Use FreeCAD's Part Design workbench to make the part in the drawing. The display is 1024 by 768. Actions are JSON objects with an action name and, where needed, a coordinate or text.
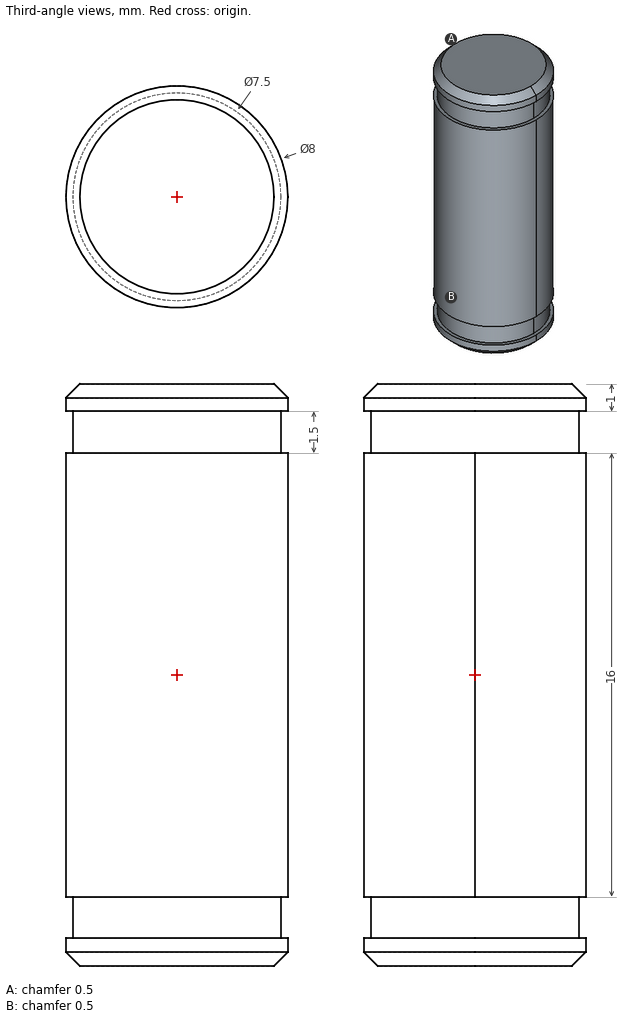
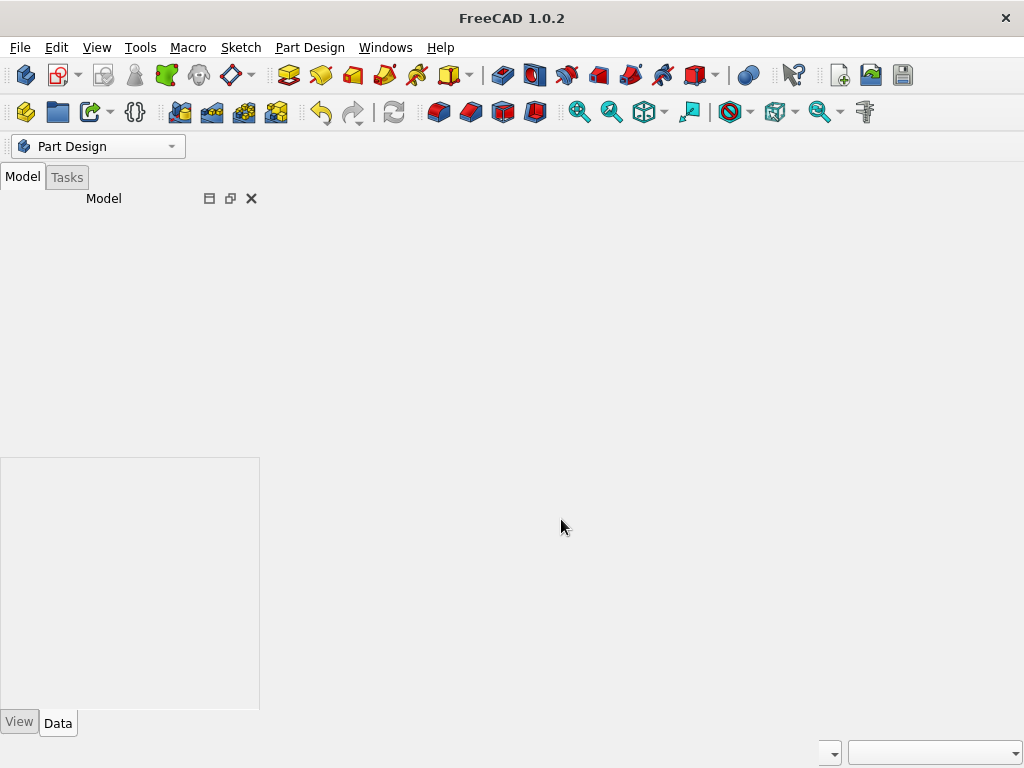
{"action": "left_click", "coordinate": [840, 76]}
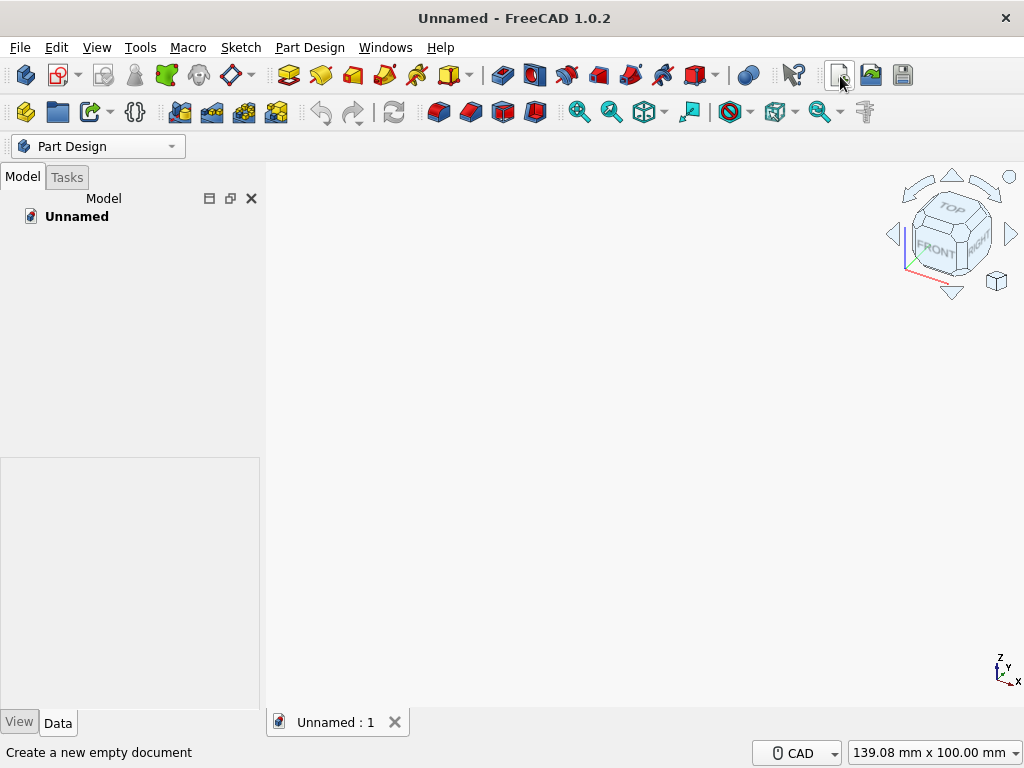
{"action": "left_click", "coordinate": [58, 76]}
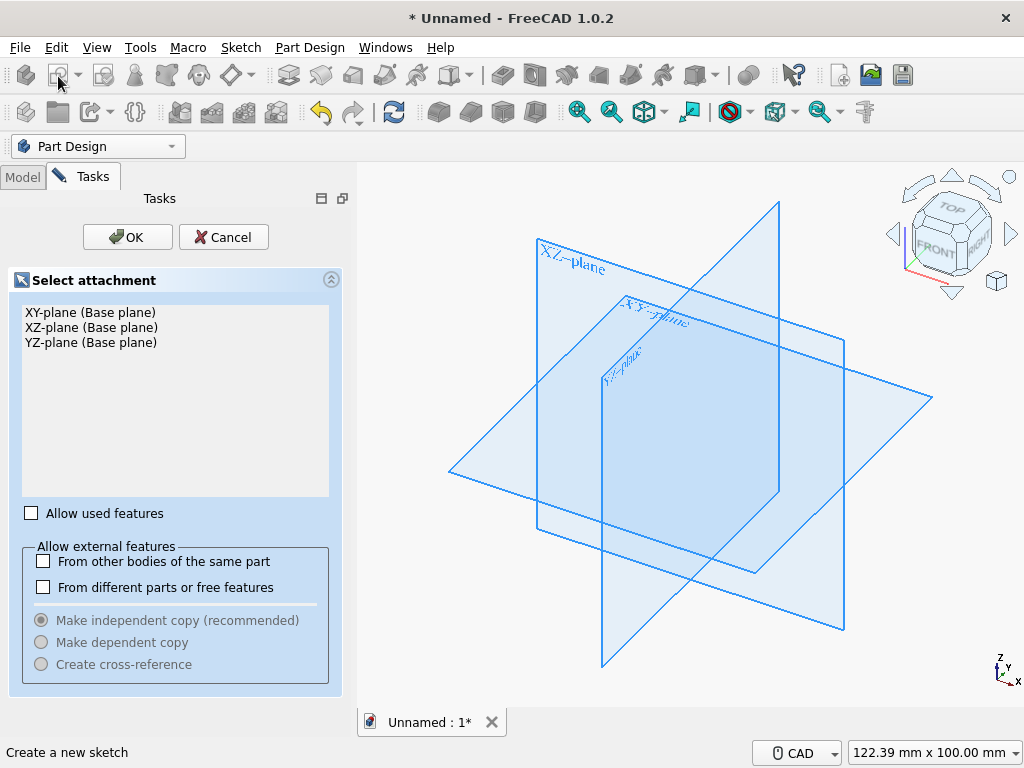
{"action": "left_click", "coordinate": [82, 312]}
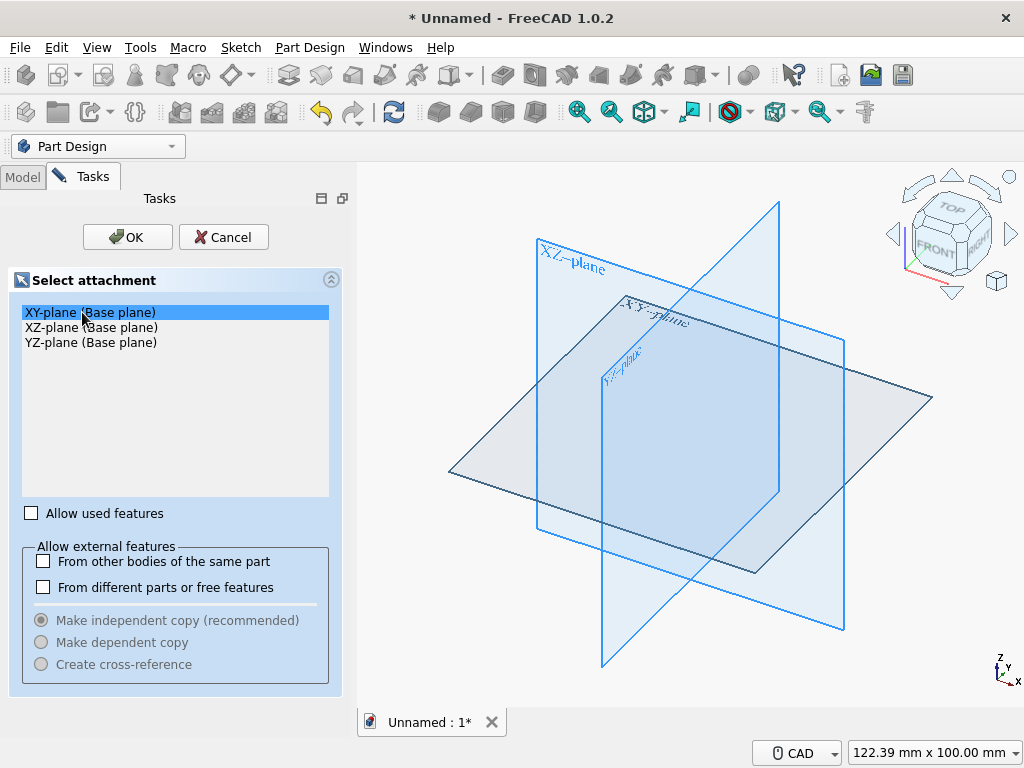
{"action": "left_click", "coordinate": [128, 237]}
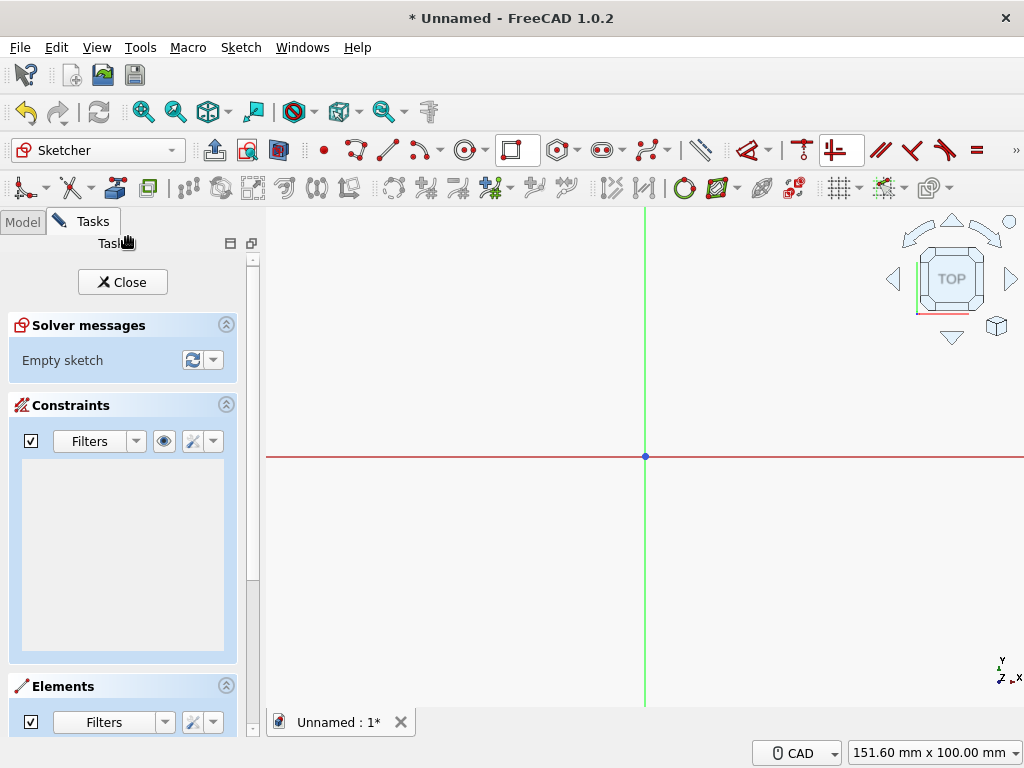
{"action": "scroll", "coordinate": [656, 457], "scroll_direction": "up", "scroll_amount": 10}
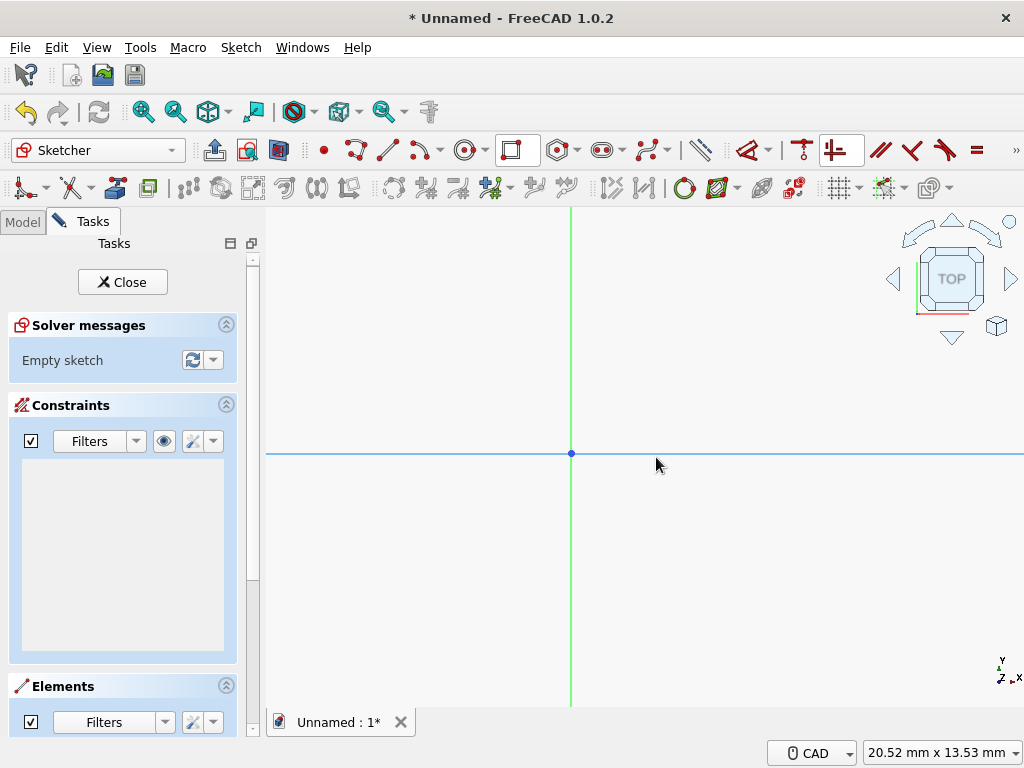
{"action": "left_click", "coordinate": [466, 150]}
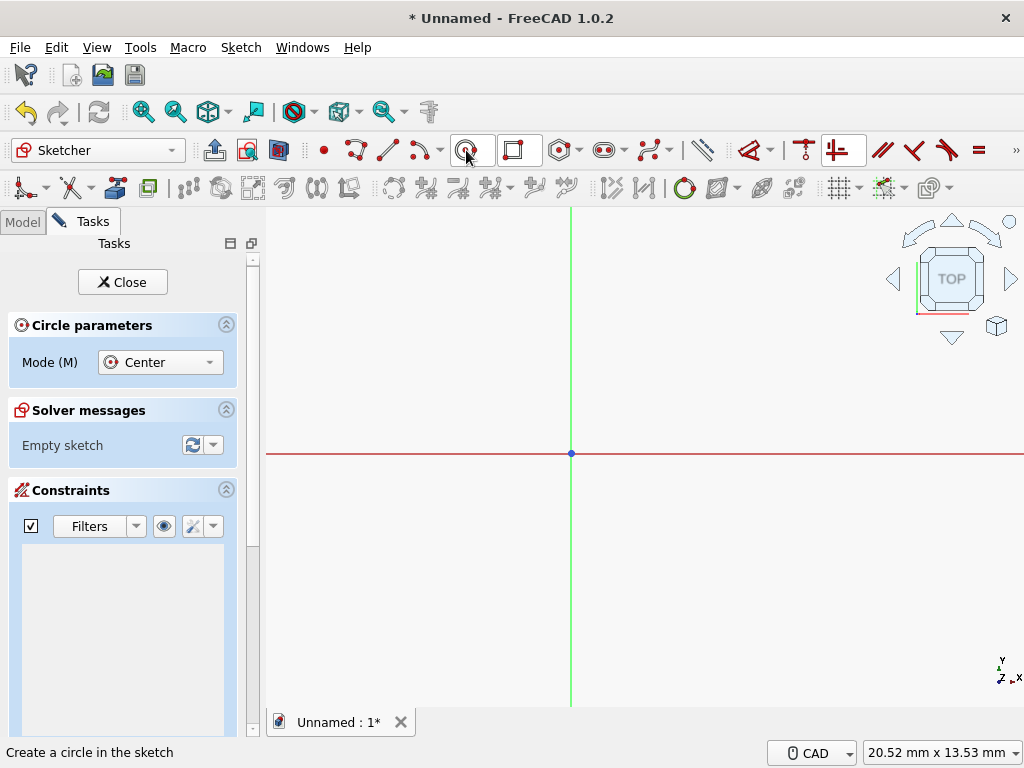
{"action": "left_click", "coordinate": [571, 454]}
{"action": "left_click", "coordinate": [676, 349]}
{"action": "key", "text": "Escape"}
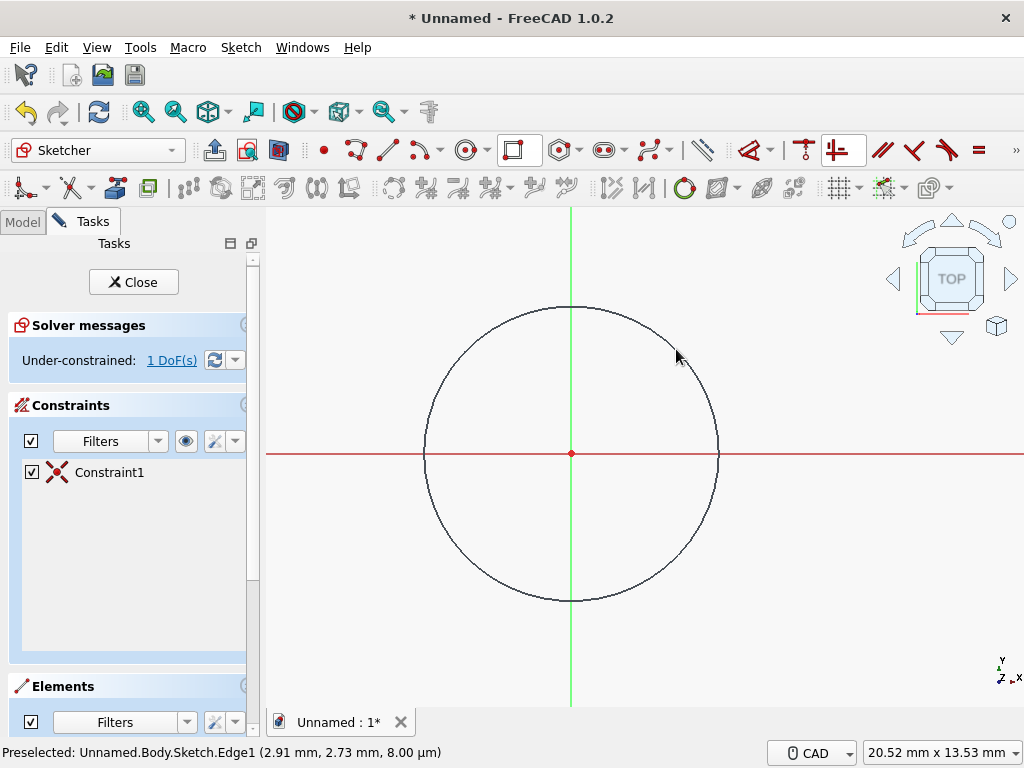
{"action": "left_click", "coordinate": [675, 349]}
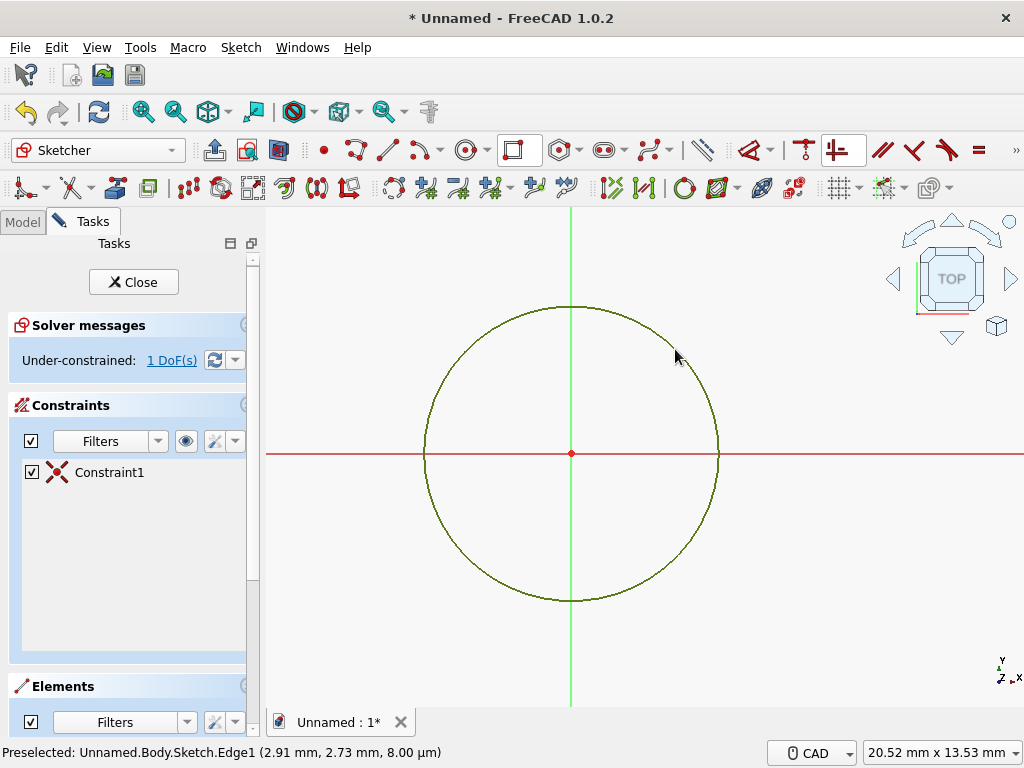
{"action": "left_click", "coordinate": [772, 150]}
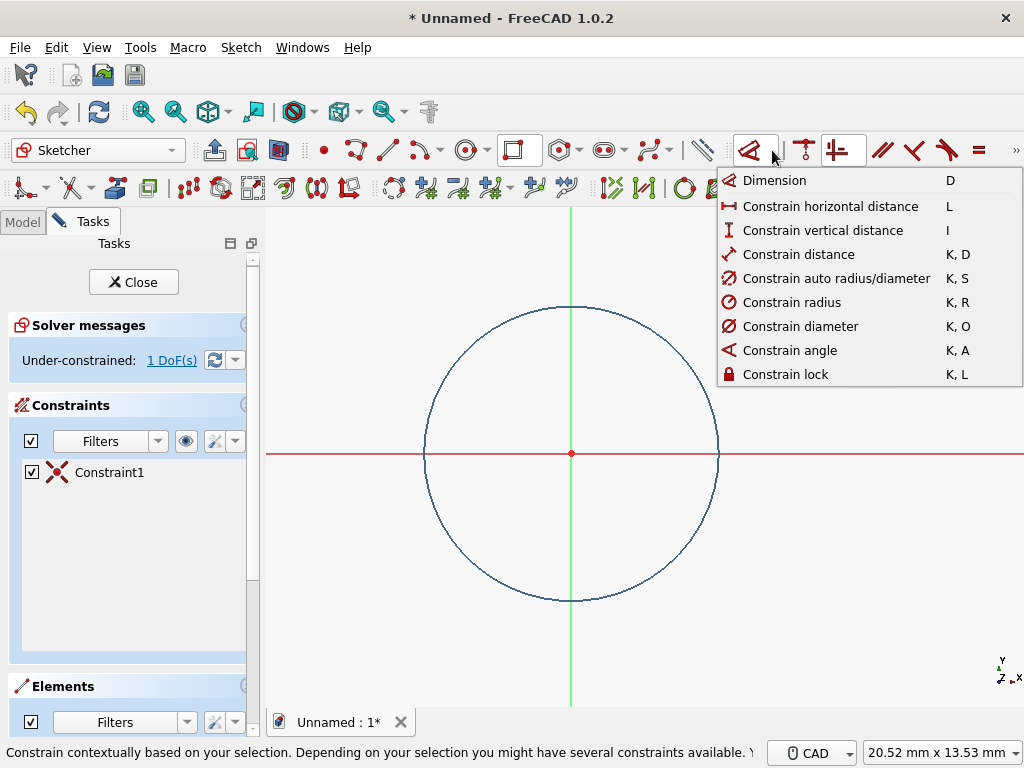
{"action": "left_click", "coordinate": [870, 326]}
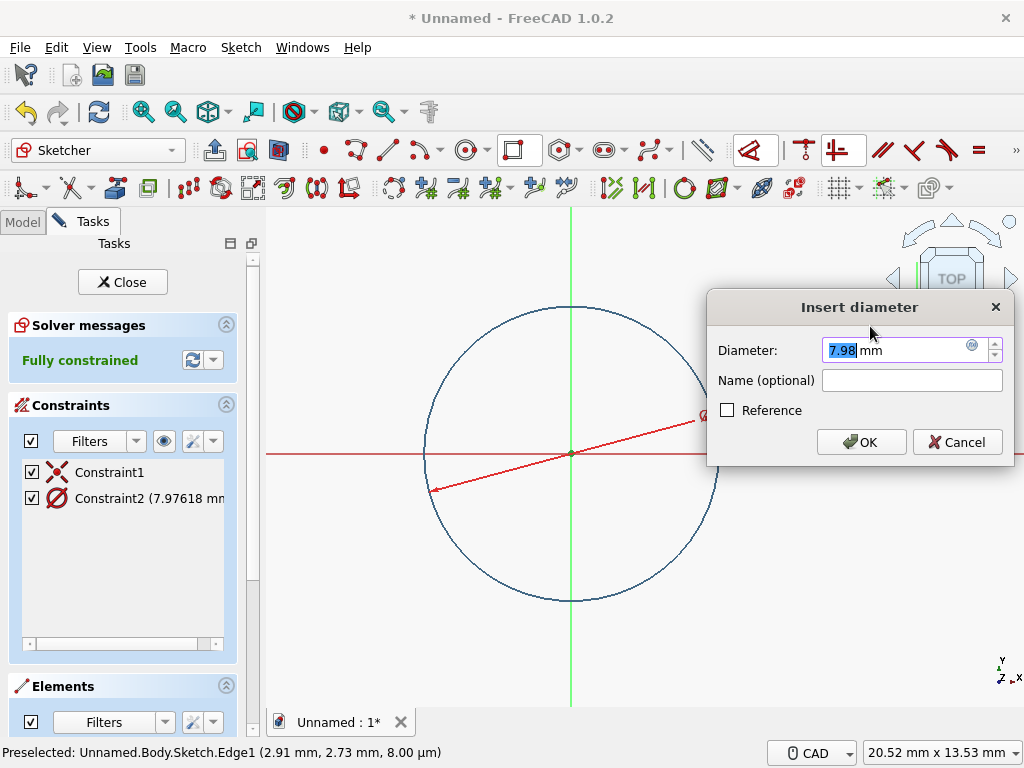
{"action": "type", "text": "8"}
{"action": "key", "text": "Return"}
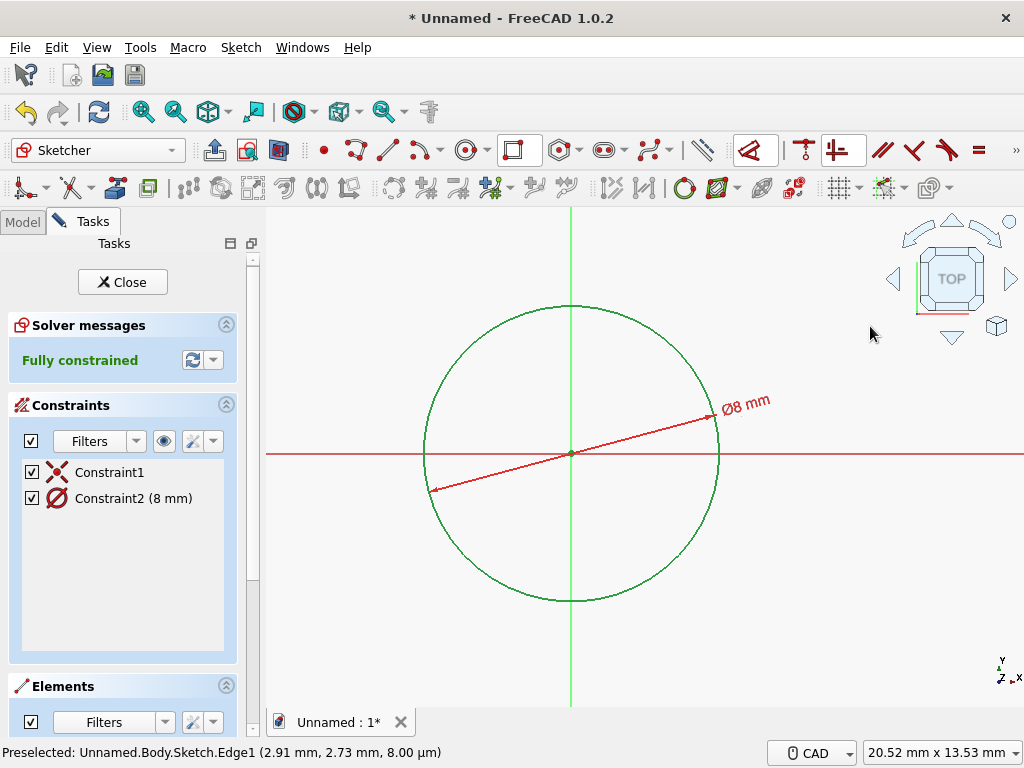
{"action": "left_click", "coordinate": [123, 282]}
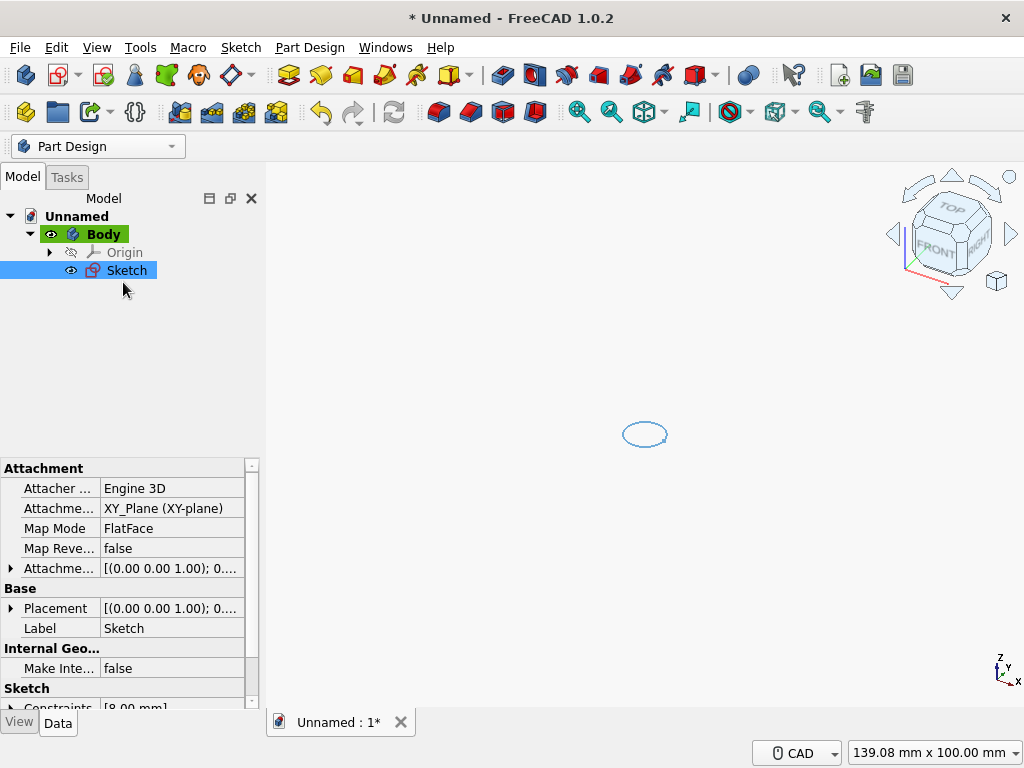
{"action": "left_click", "coordinate": [290, 76]}